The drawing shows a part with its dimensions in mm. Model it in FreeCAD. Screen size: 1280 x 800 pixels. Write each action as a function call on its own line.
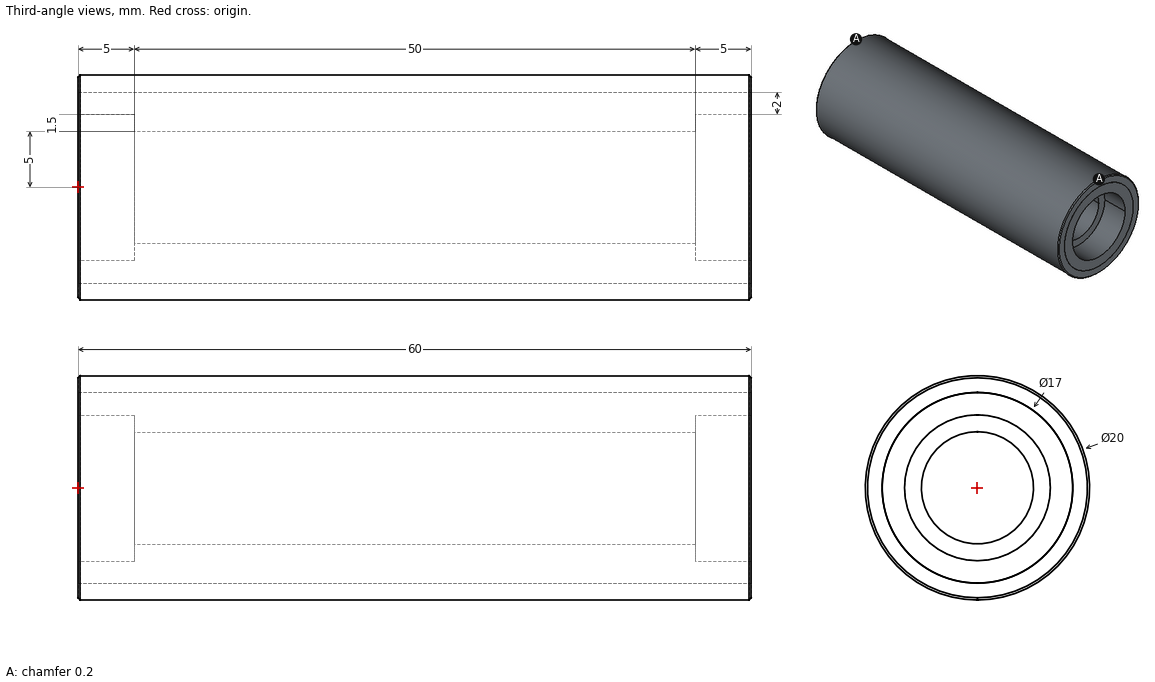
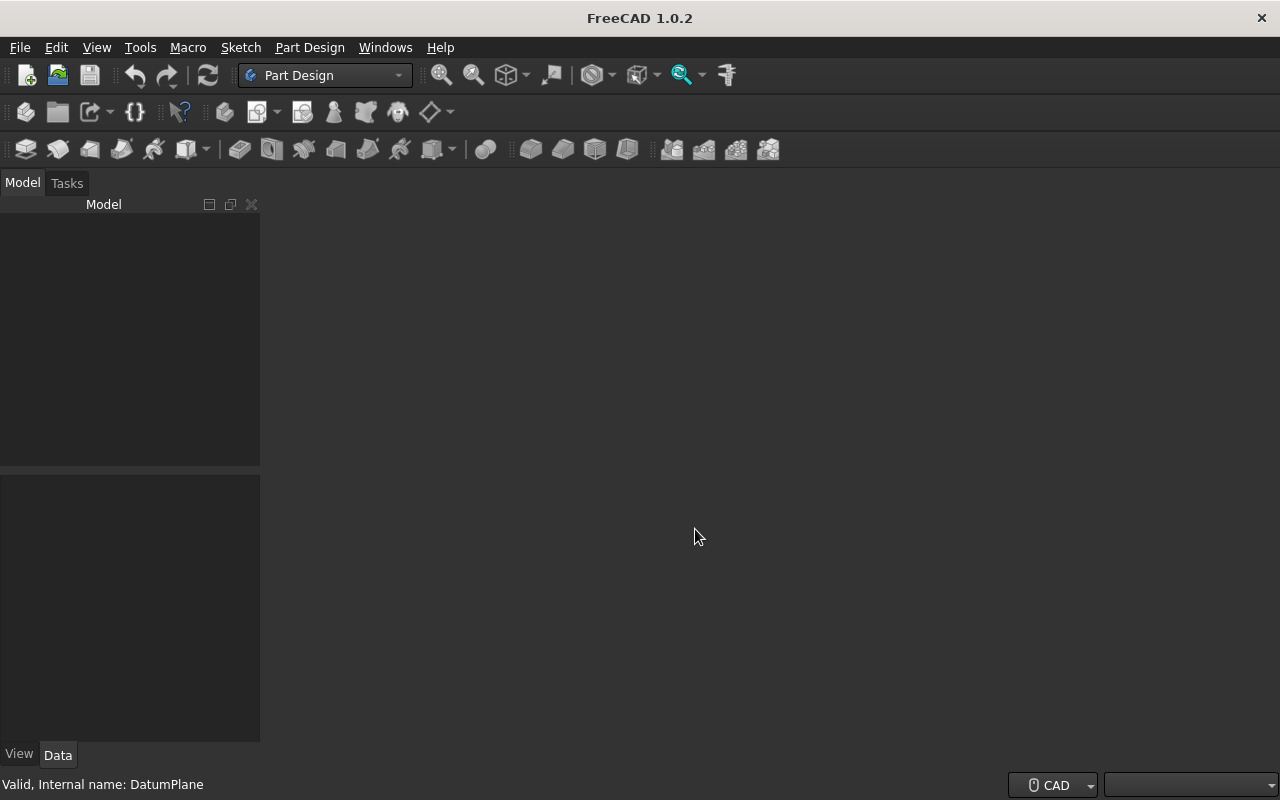
click(26, 76)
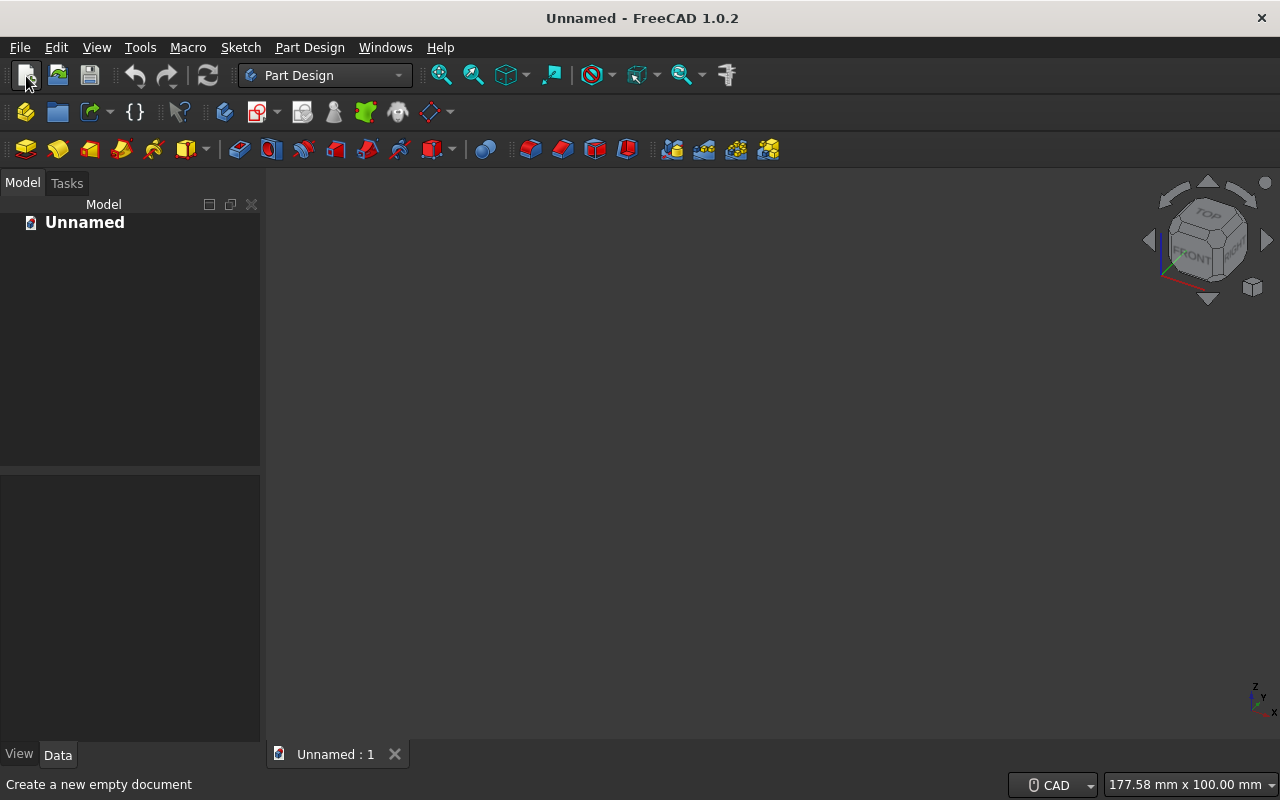
click(258, 112)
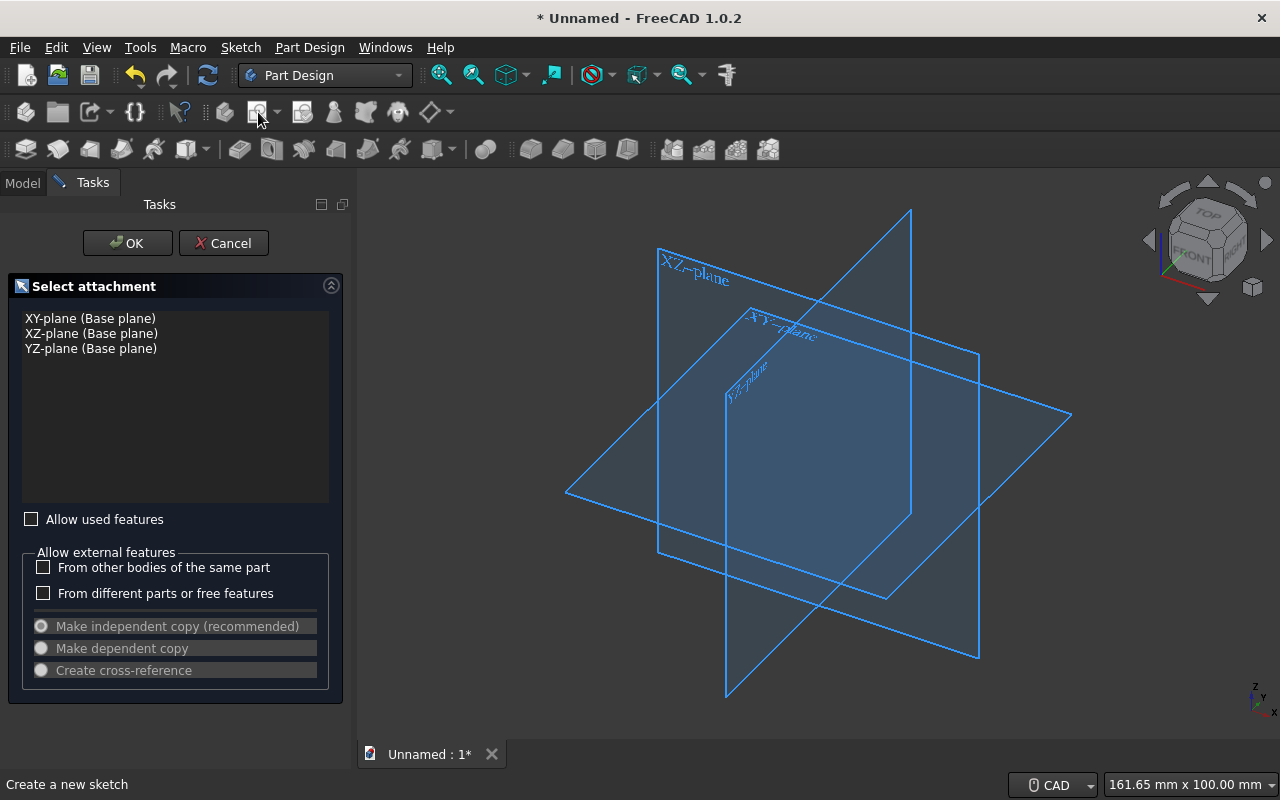
click(82, 318)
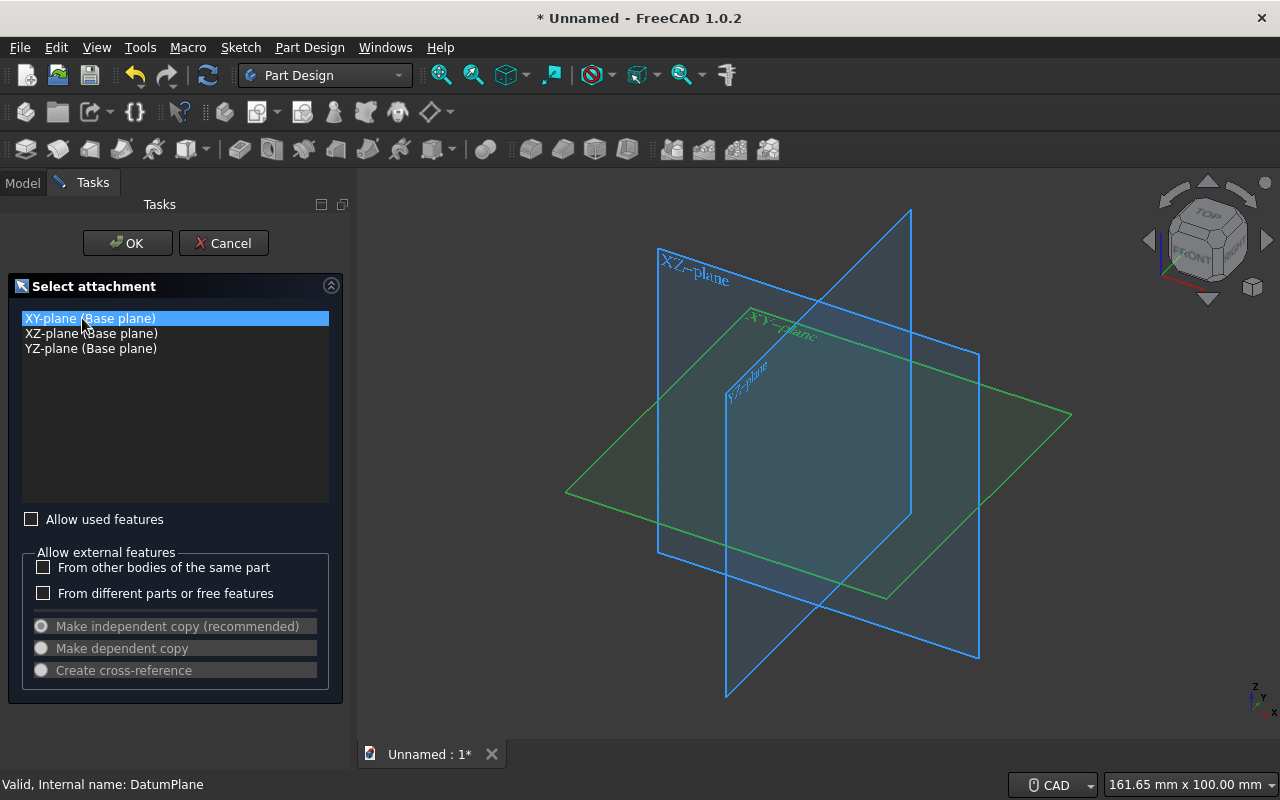
click(128, 243)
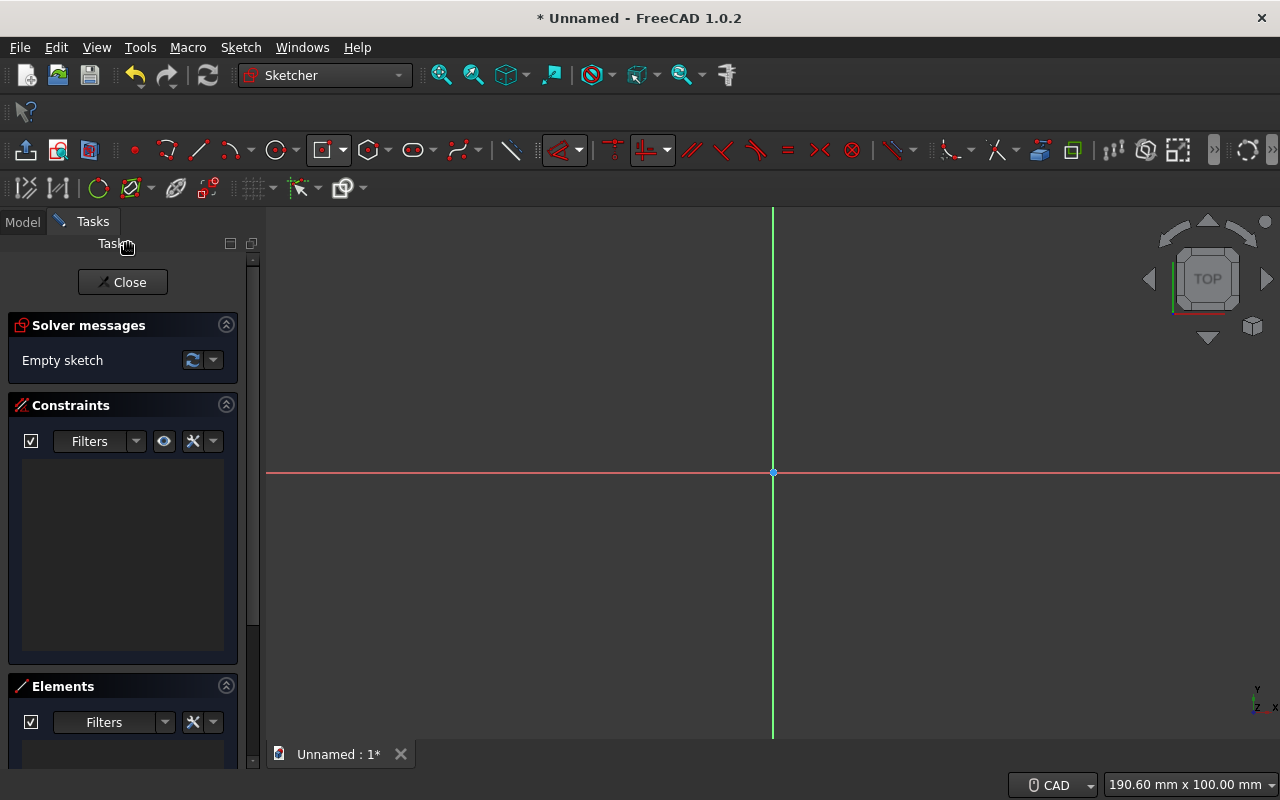
scroll(1115, 423, up, 3)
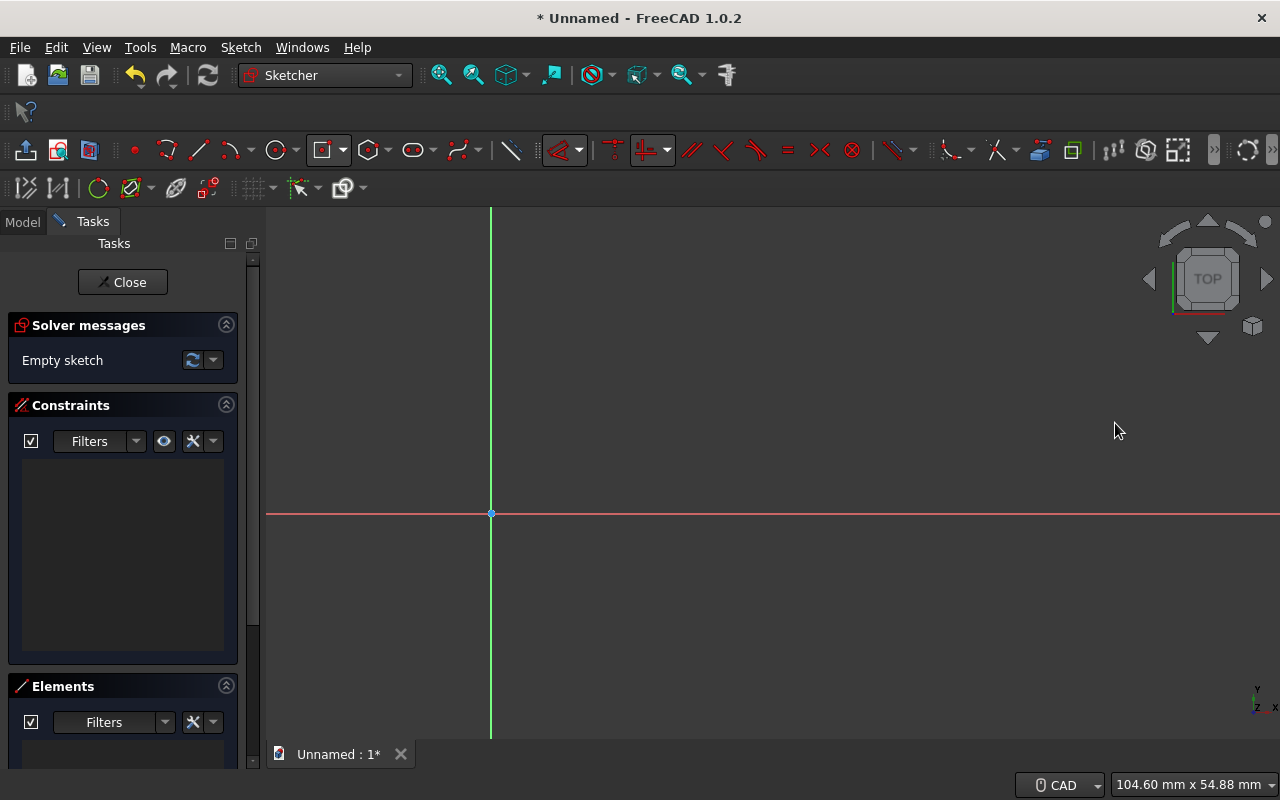
click(168, 150)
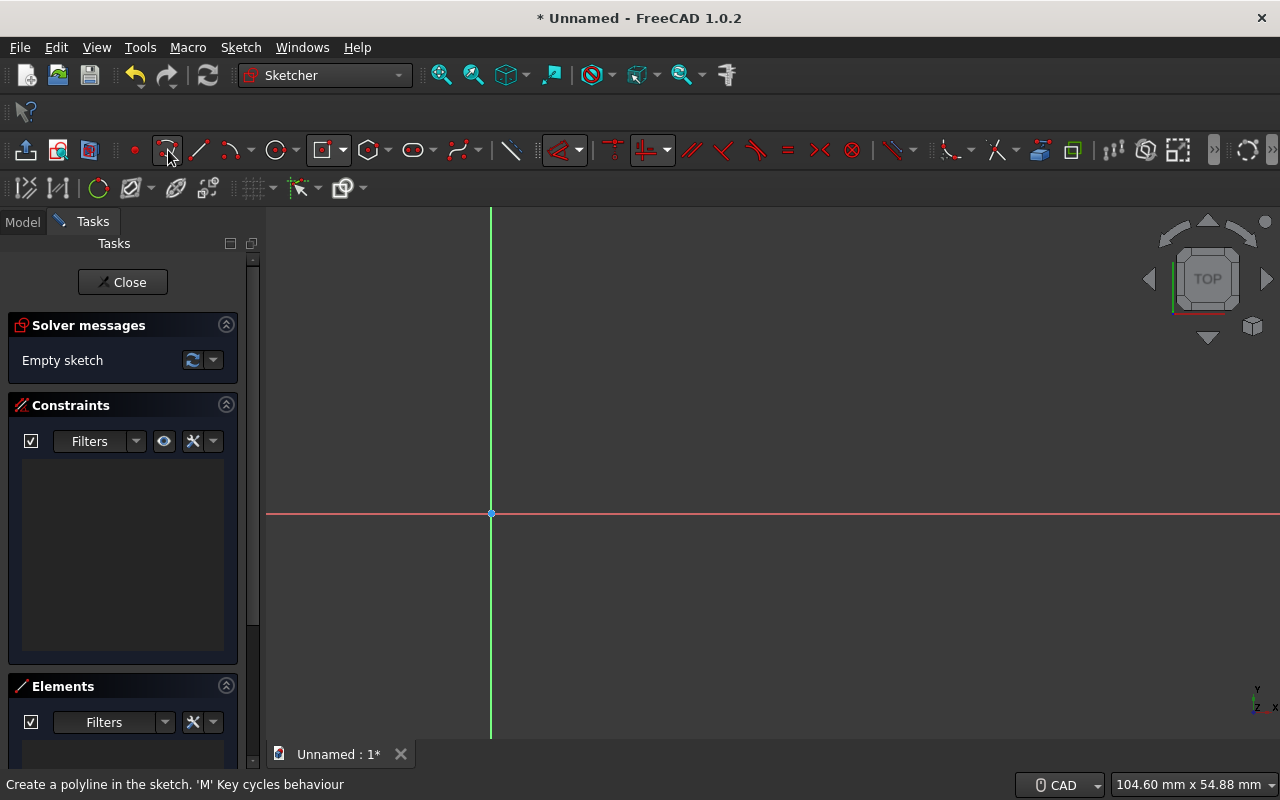
click(491, 451)
click(540, 451)
click(540, 465)
click(1024, 465)
click(1024, 451)
click(1073, 451)
click(1073, 431)
click(500, 431)
click(491, 452)
key(Escape)
key(Escape)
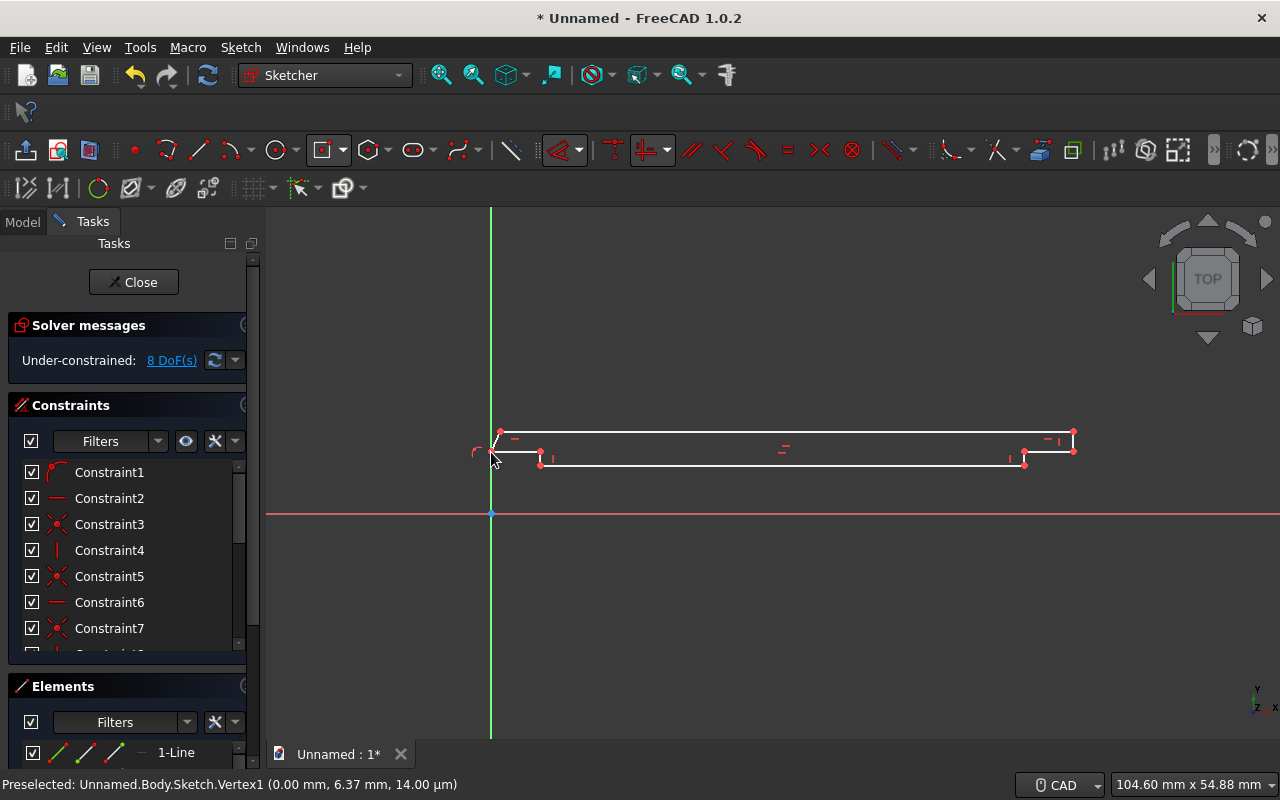
scroll(495, 444, up, 3)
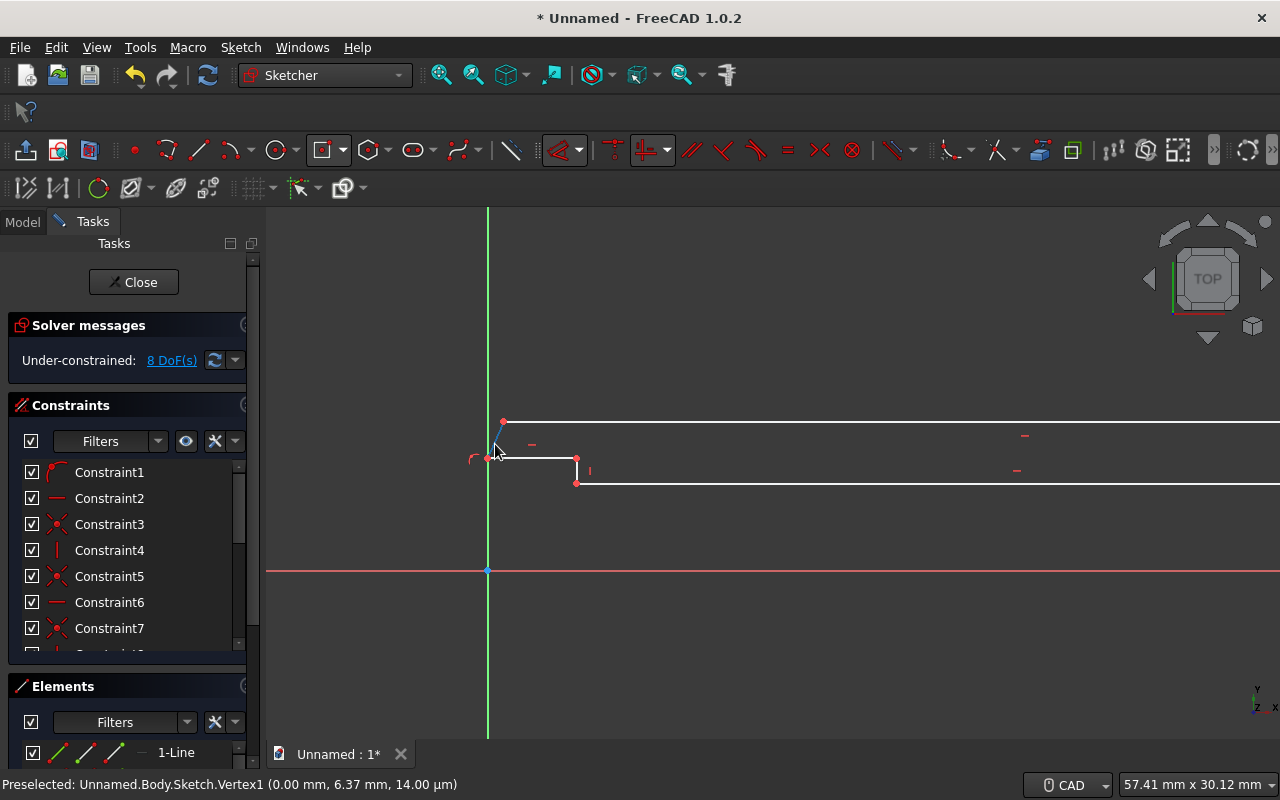
click(494, 444)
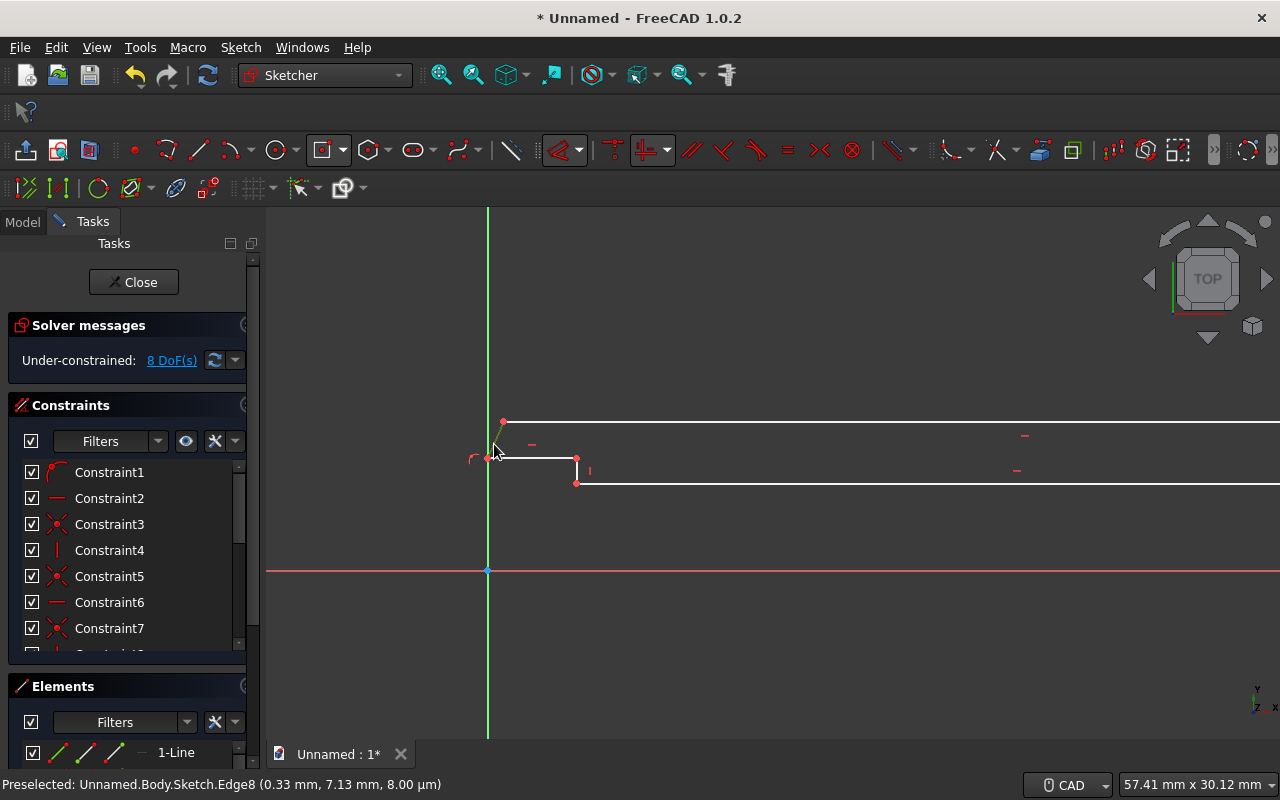
key(v)